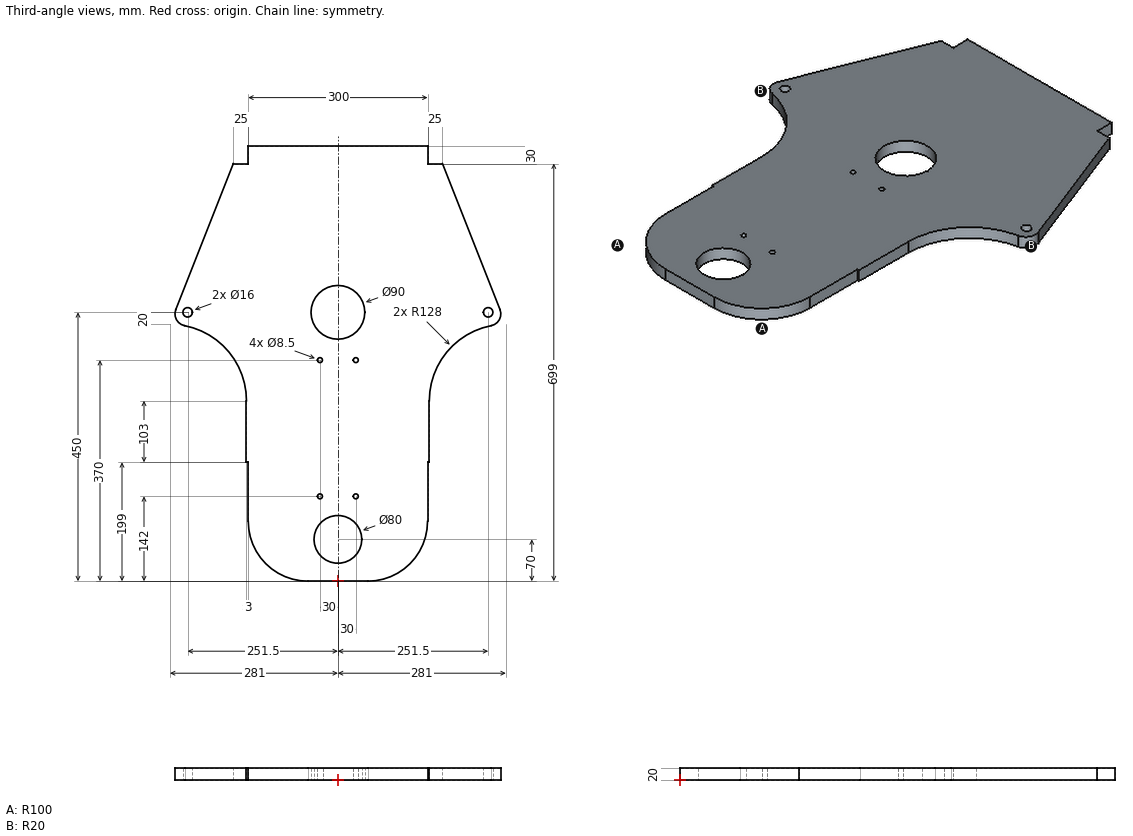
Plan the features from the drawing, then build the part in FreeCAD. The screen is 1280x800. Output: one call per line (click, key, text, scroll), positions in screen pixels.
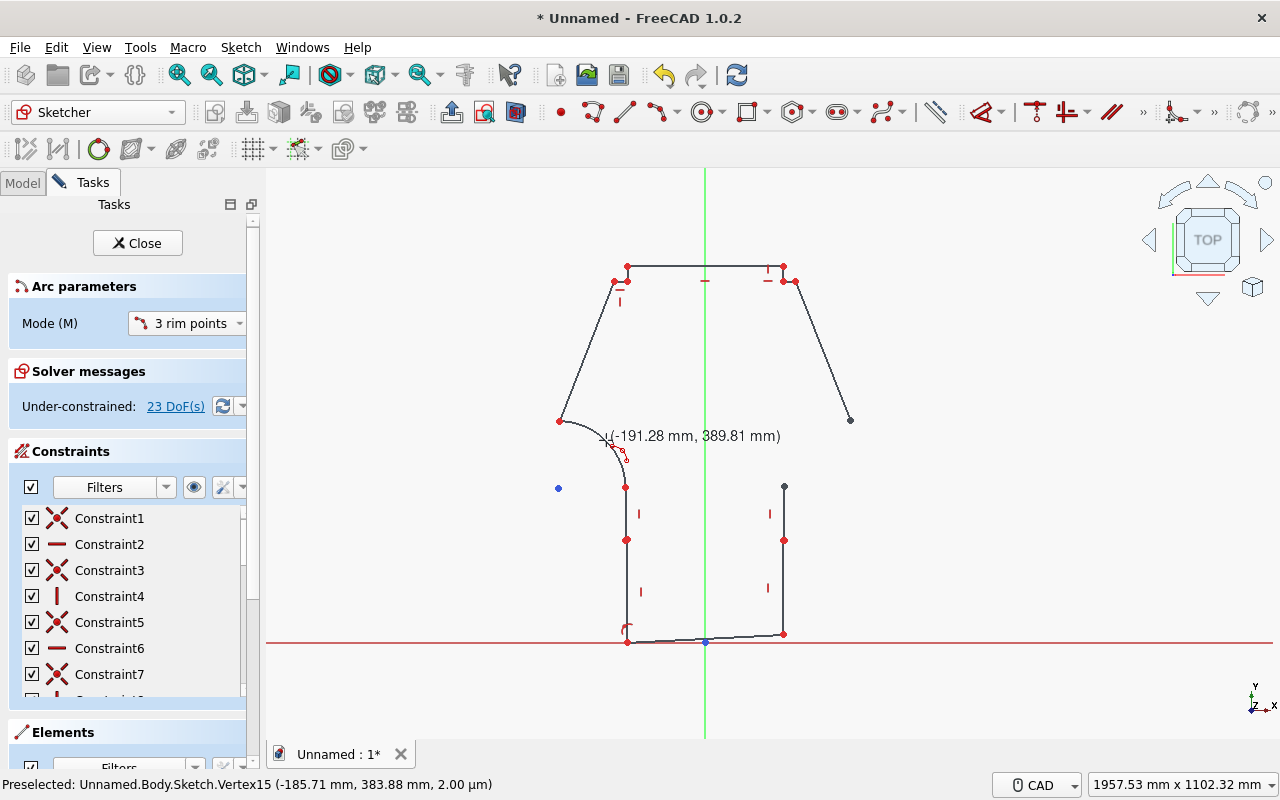
click(784, 487)
click(851, 421)
click(804, 440)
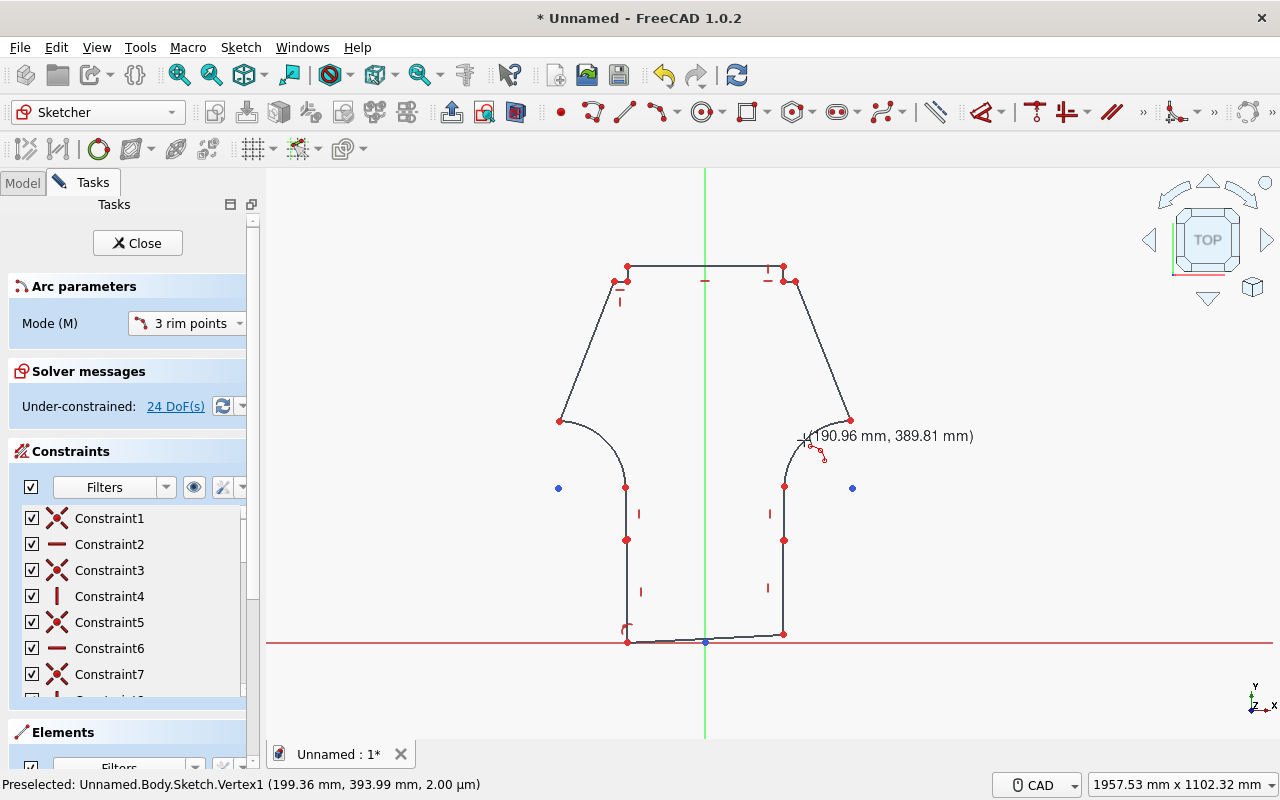
click(702, 112)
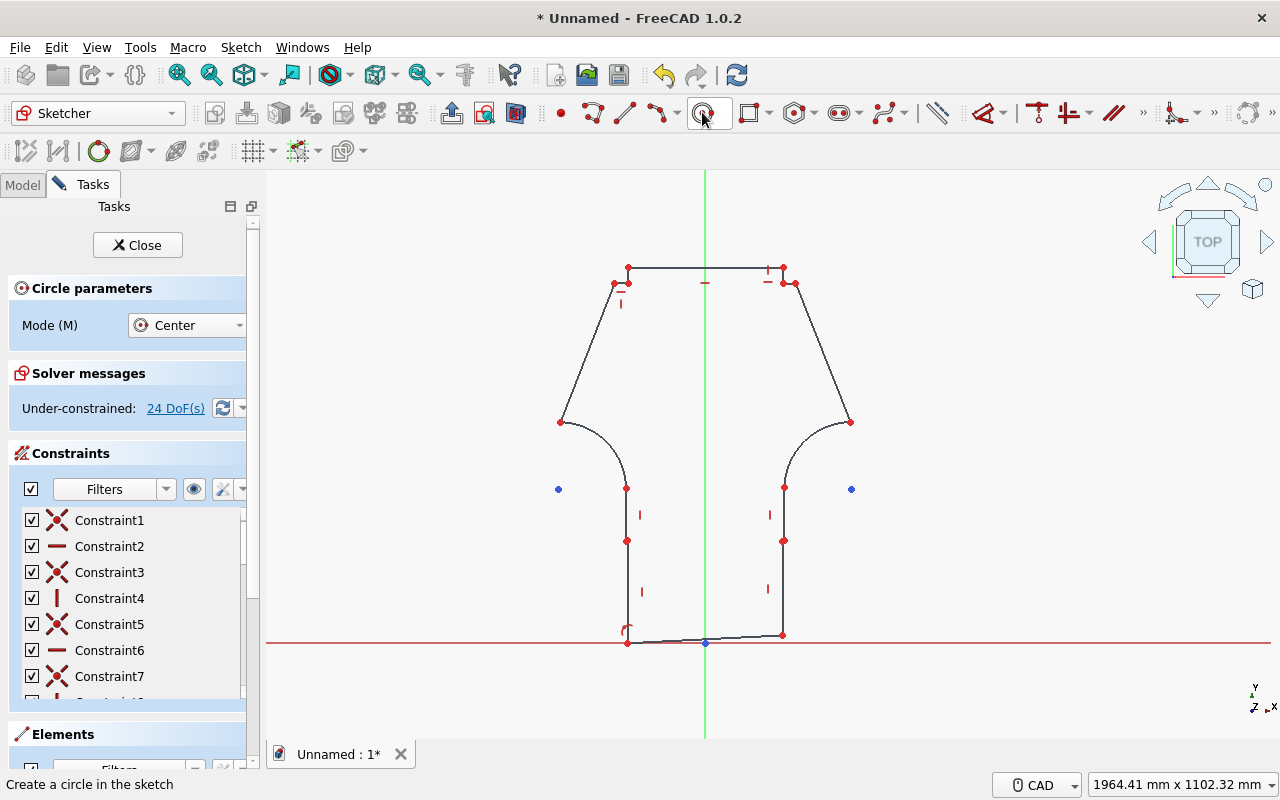
click(705, 607)
move(720, 593)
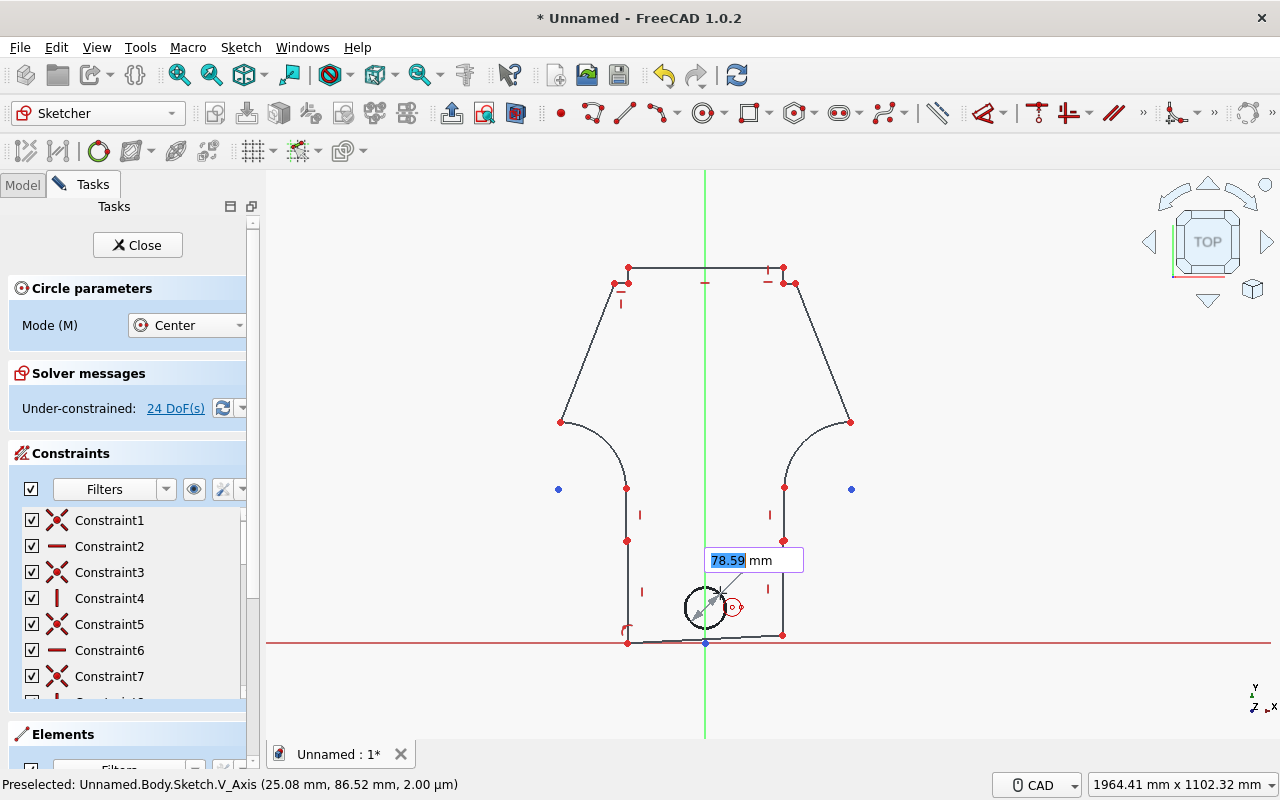
text(80)
key(Return)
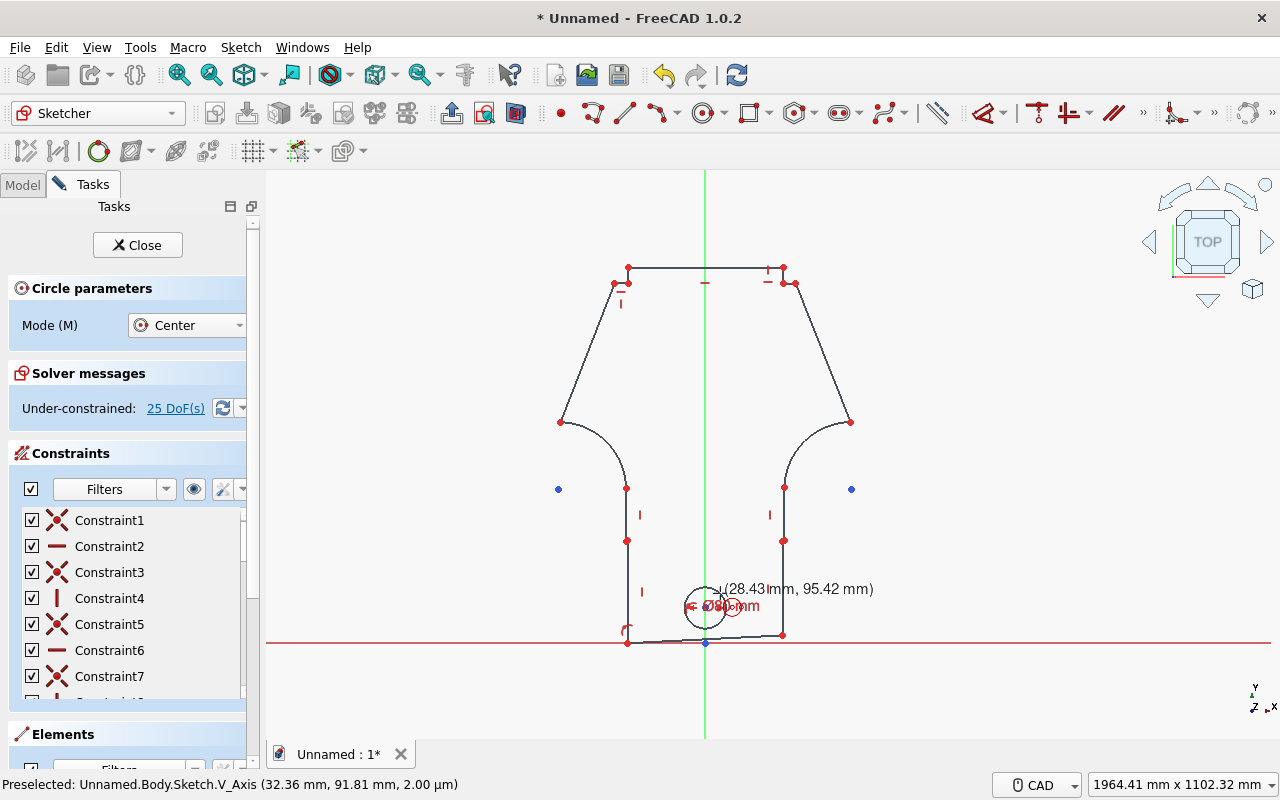
scroll(576, 411, up, 9)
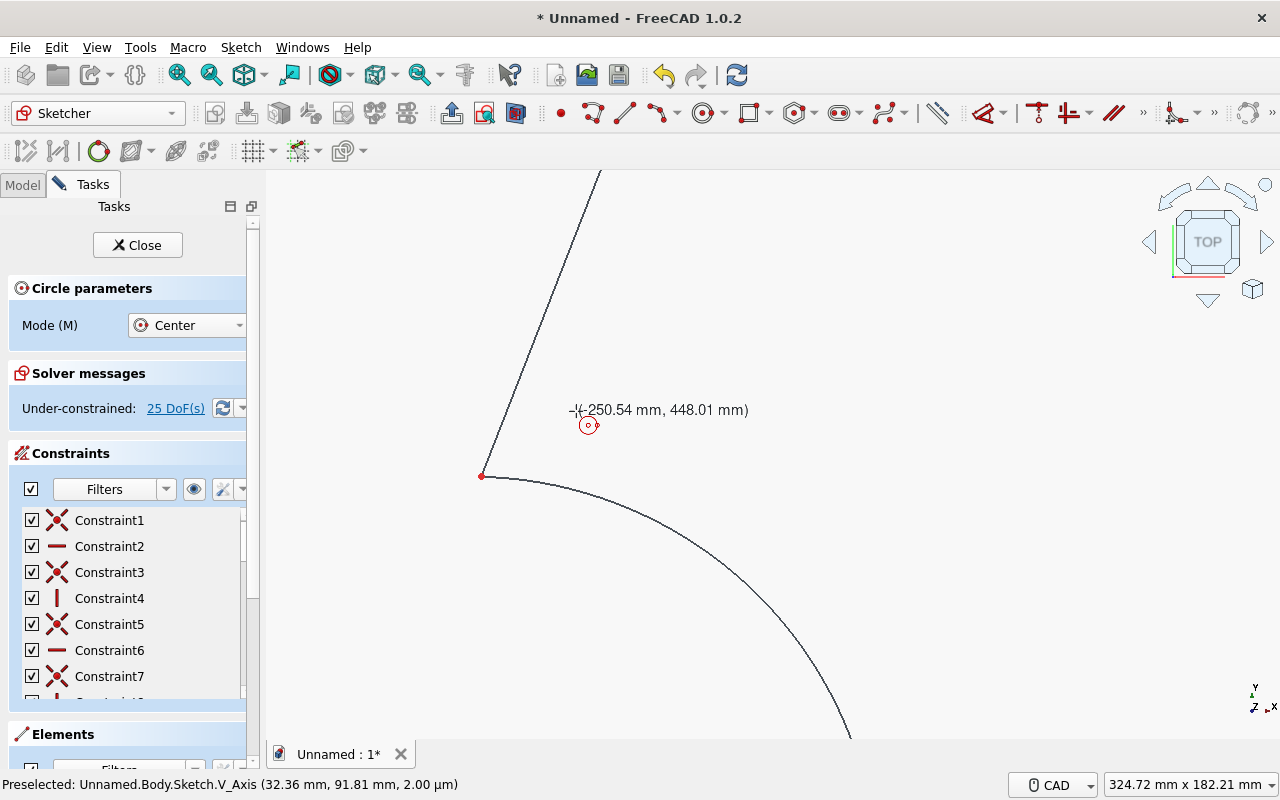
scroll(575, 411, down, 9)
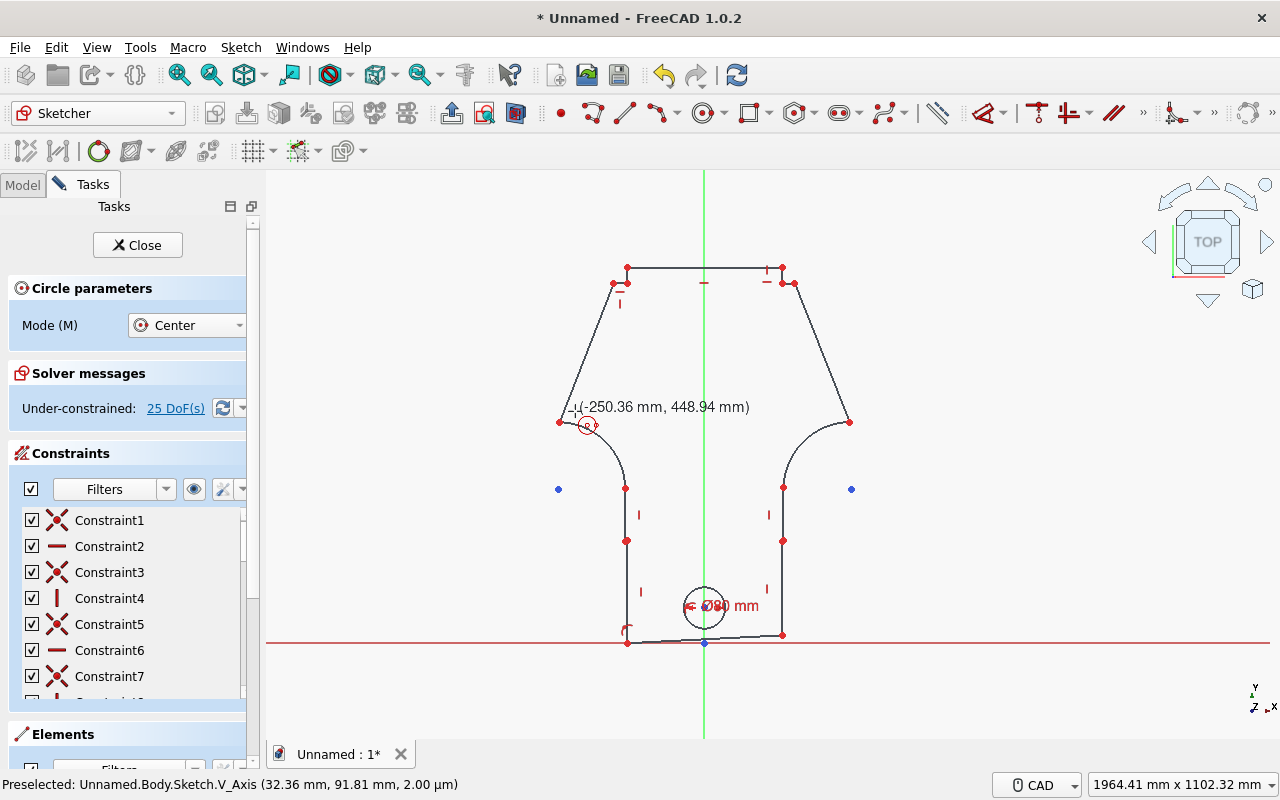
scroll(575, 411, up, 3)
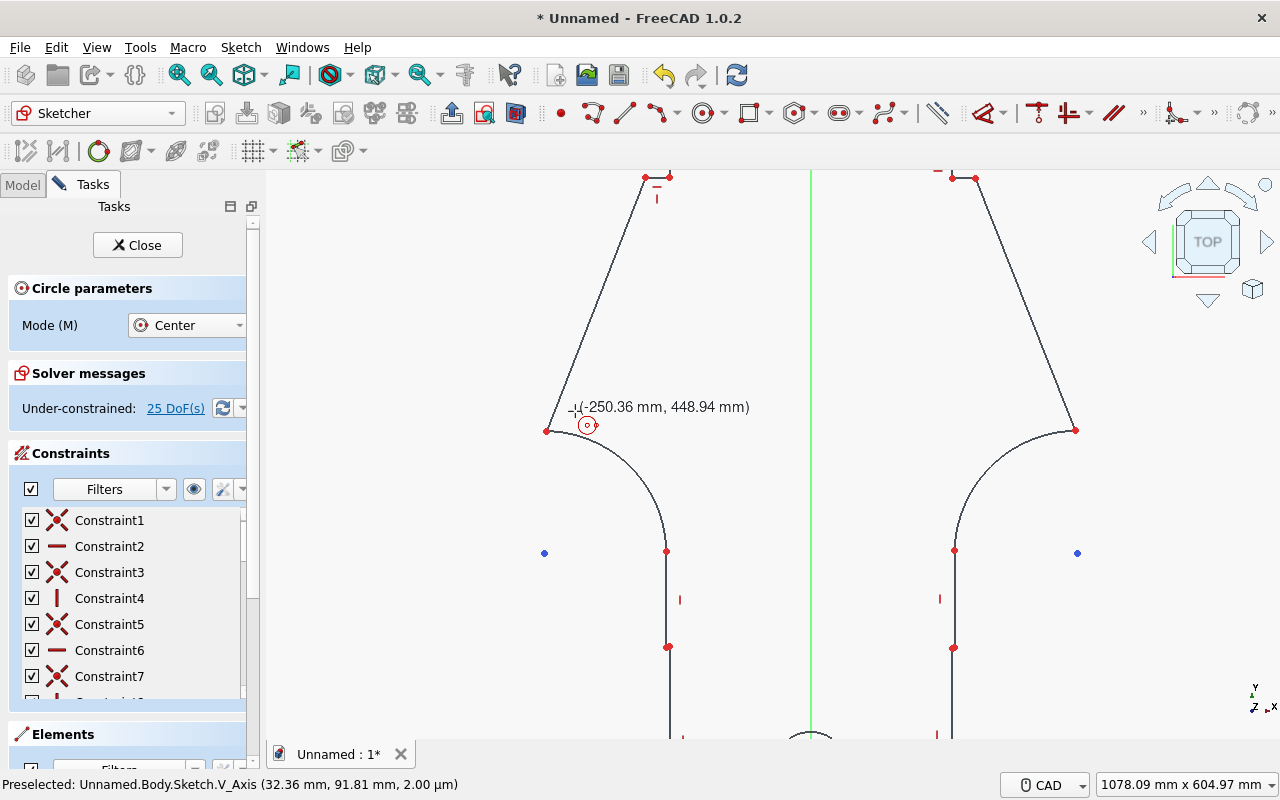
click(574, 411)
move(579, 405)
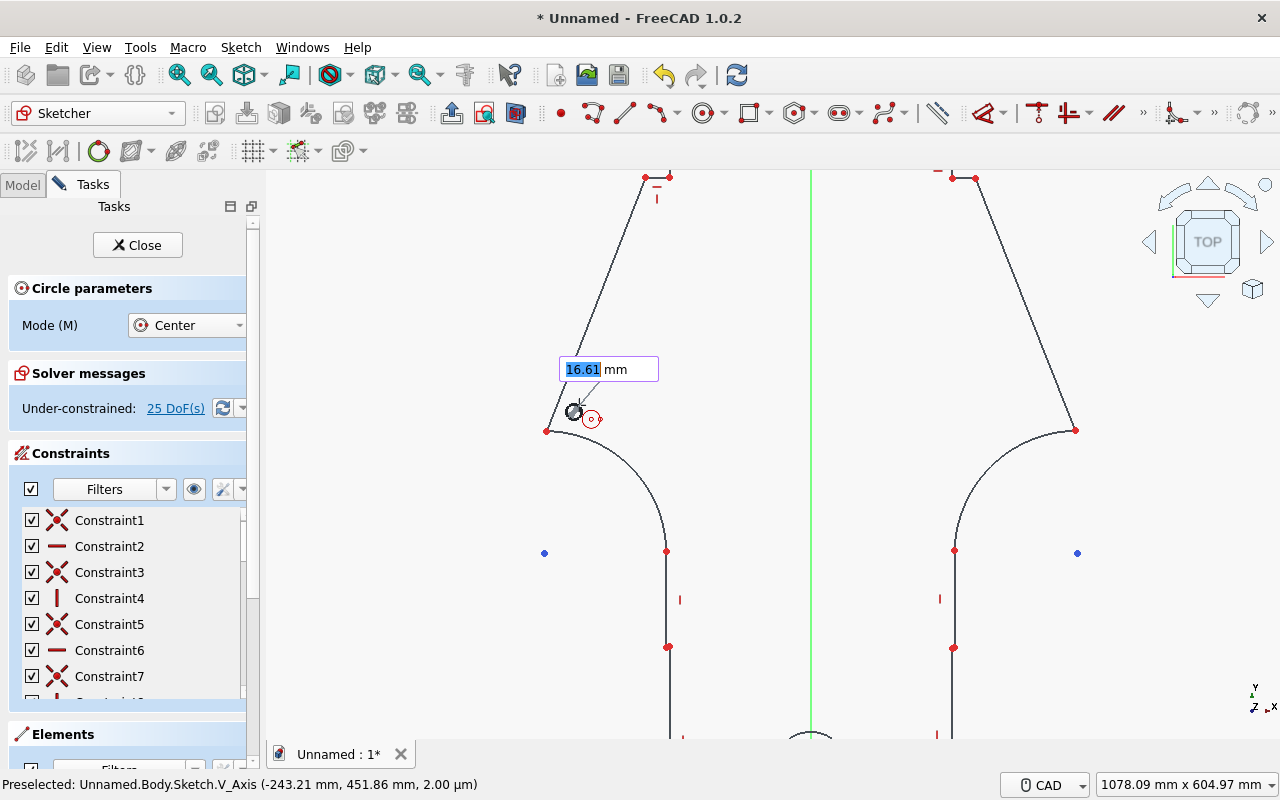
text(16)
key(Return)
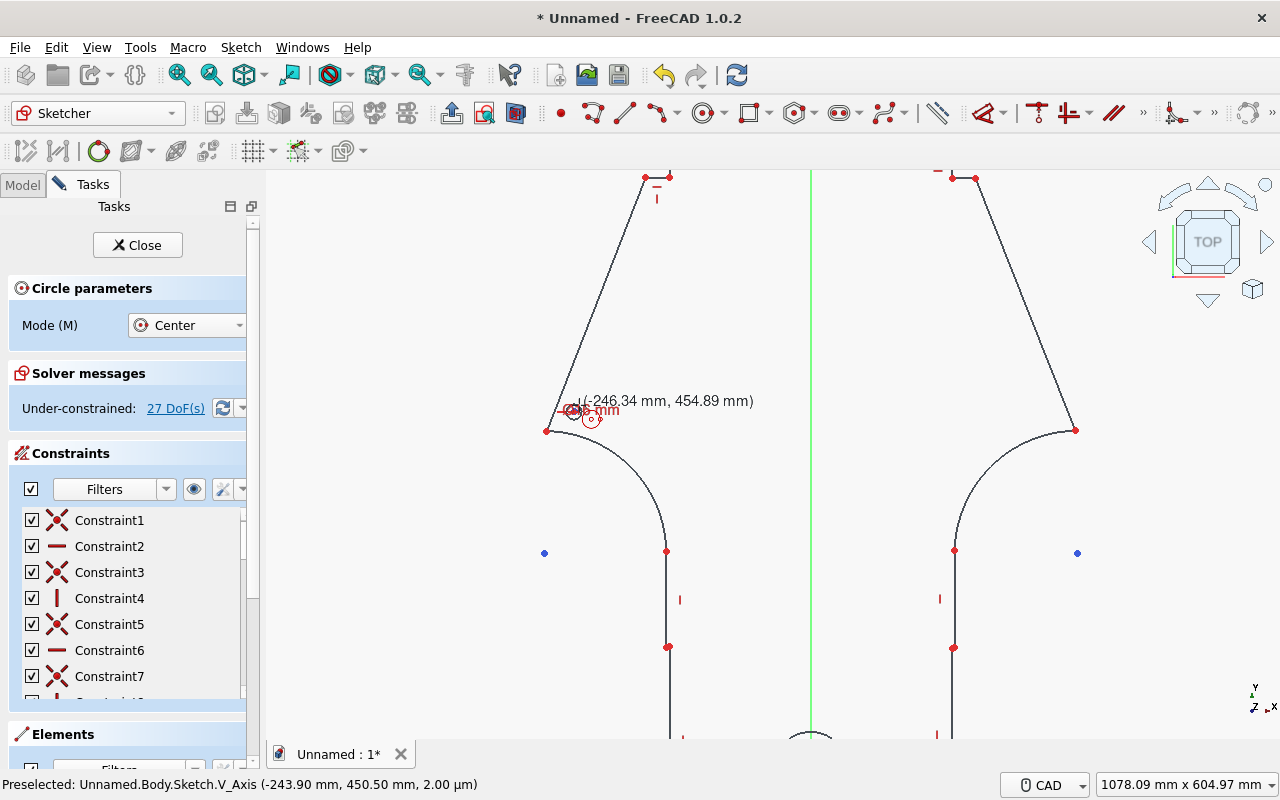
click(811, 411)
move(841, 381)